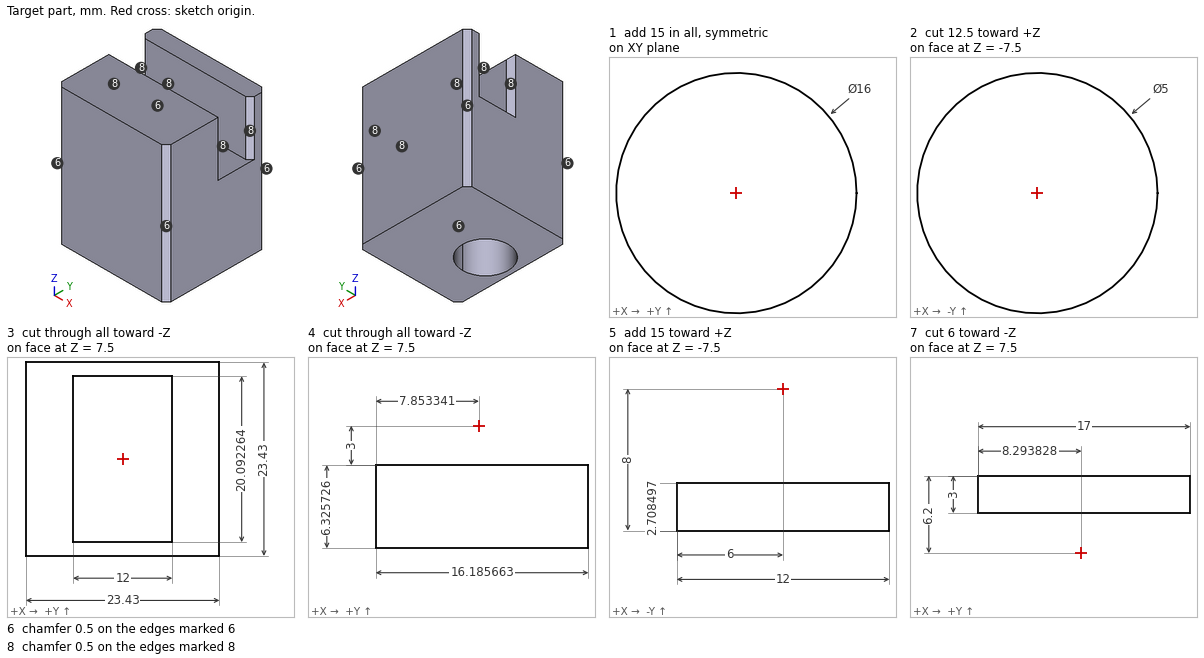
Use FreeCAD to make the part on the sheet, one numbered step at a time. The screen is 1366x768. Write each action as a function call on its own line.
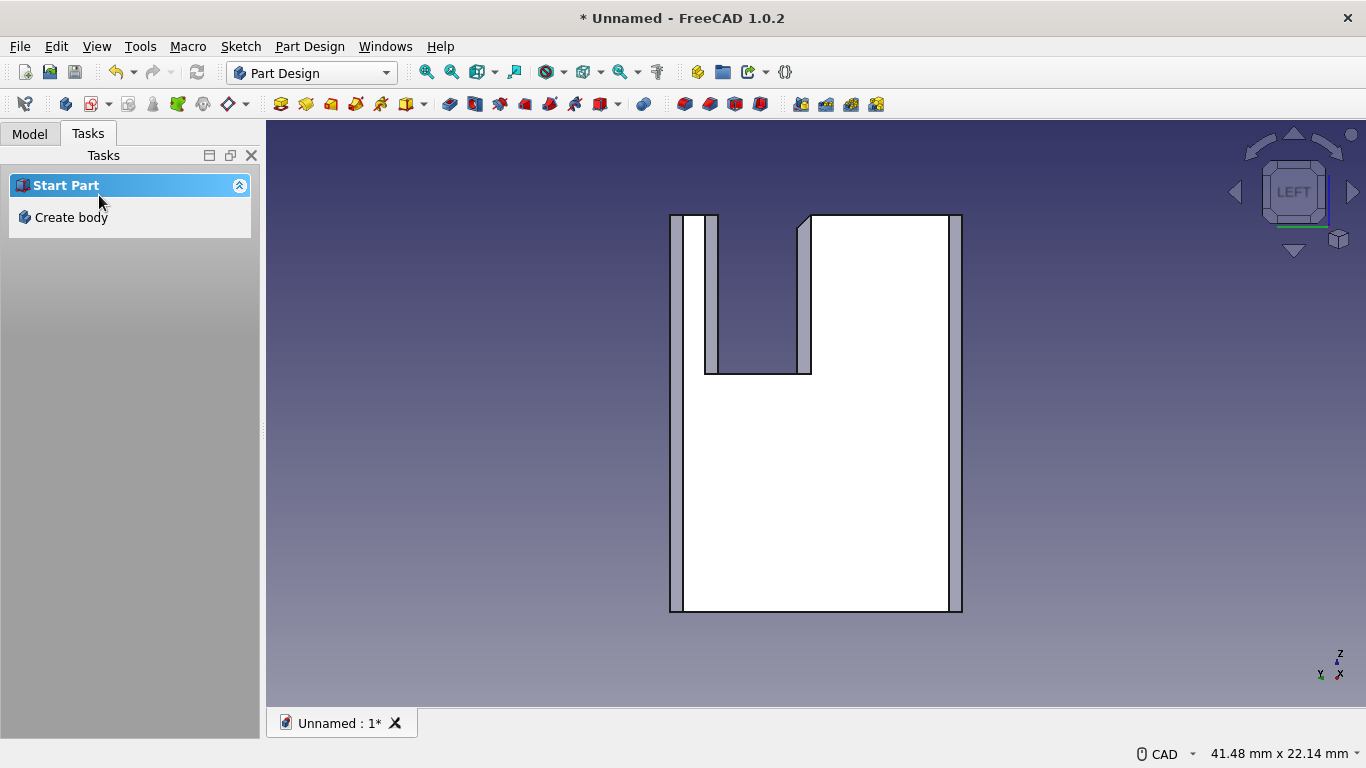
key(0)